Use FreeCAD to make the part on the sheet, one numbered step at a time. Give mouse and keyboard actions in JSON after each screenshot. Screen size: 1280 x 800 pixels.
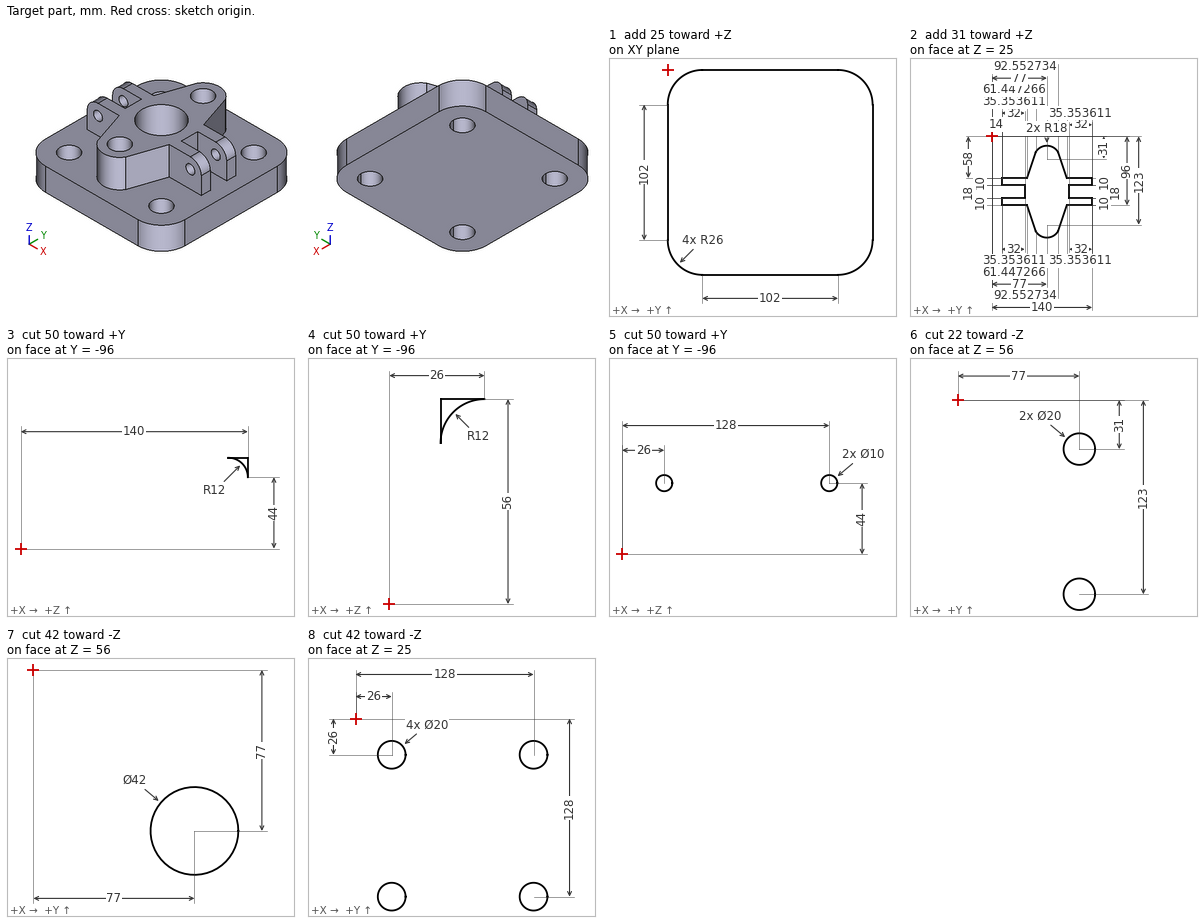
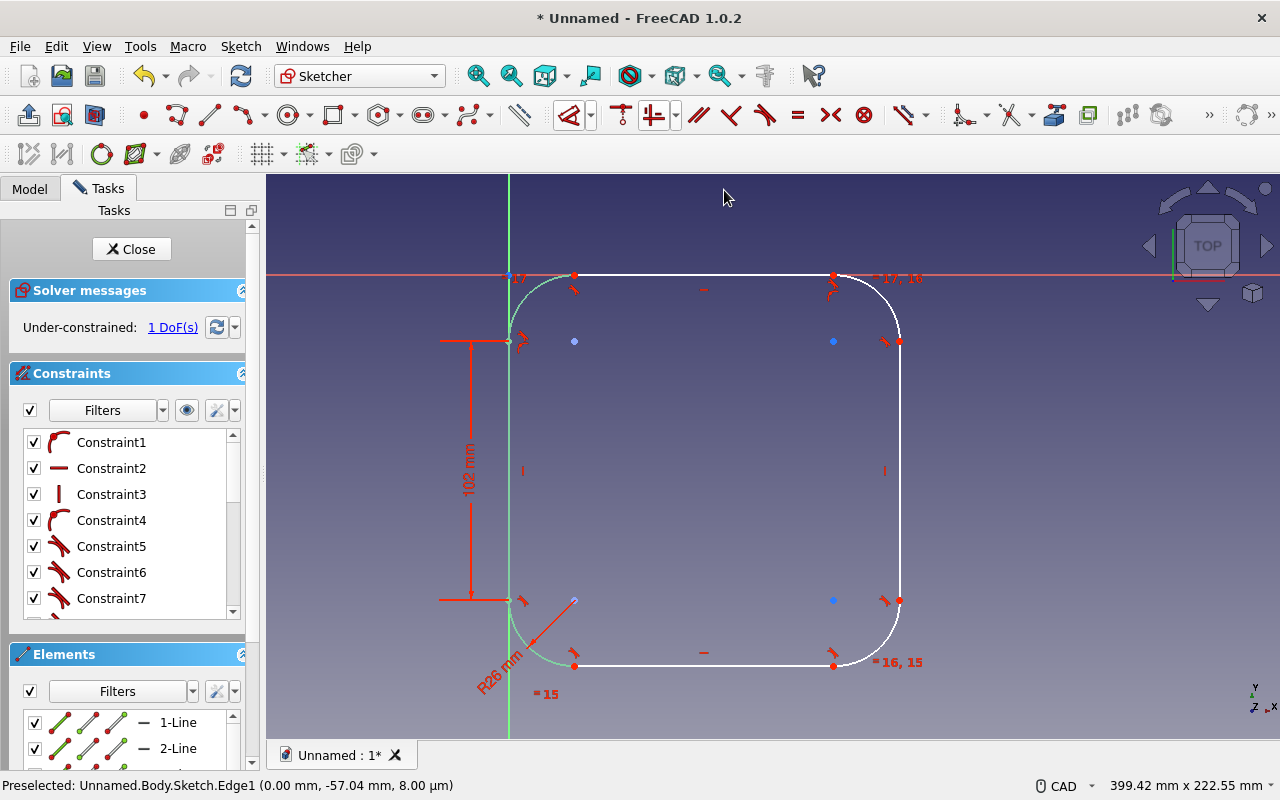
{"action": "left_click", "coordinate": [653, 666]}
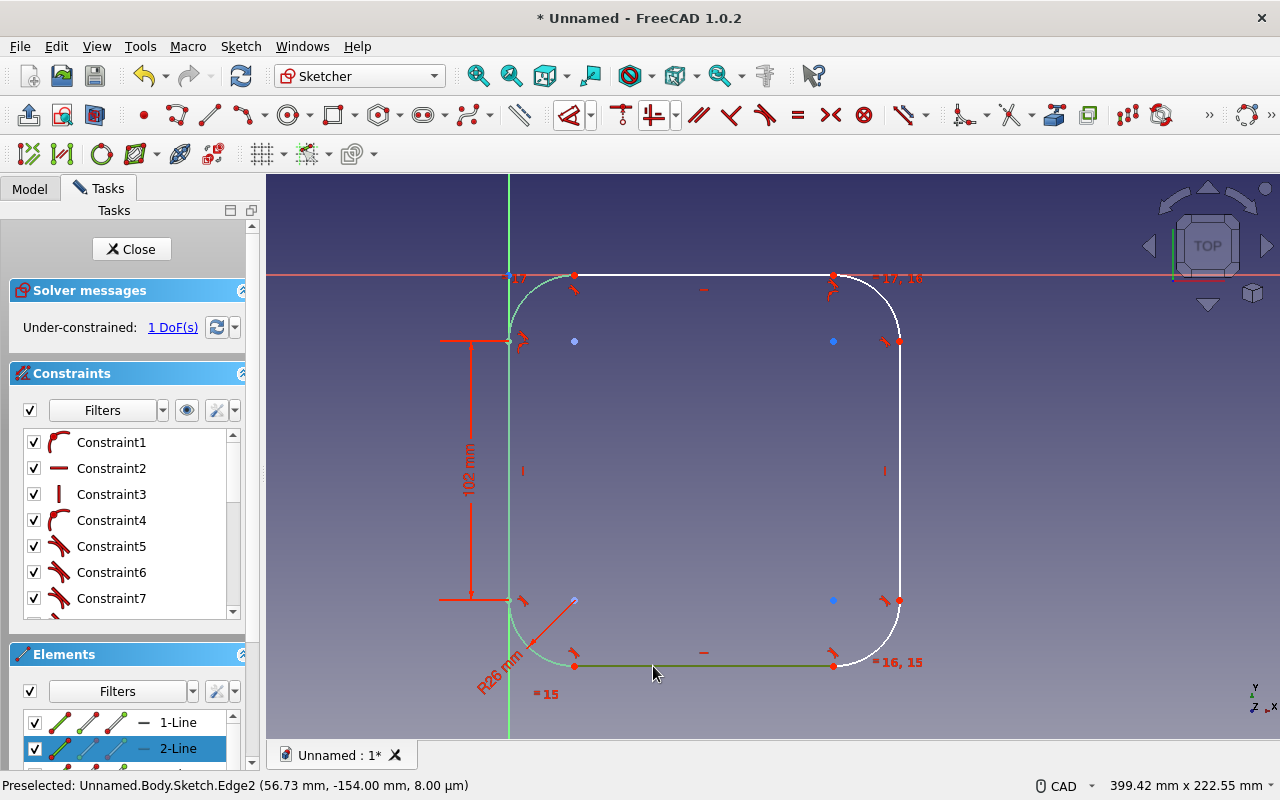
{"action": "key", "text": "l"}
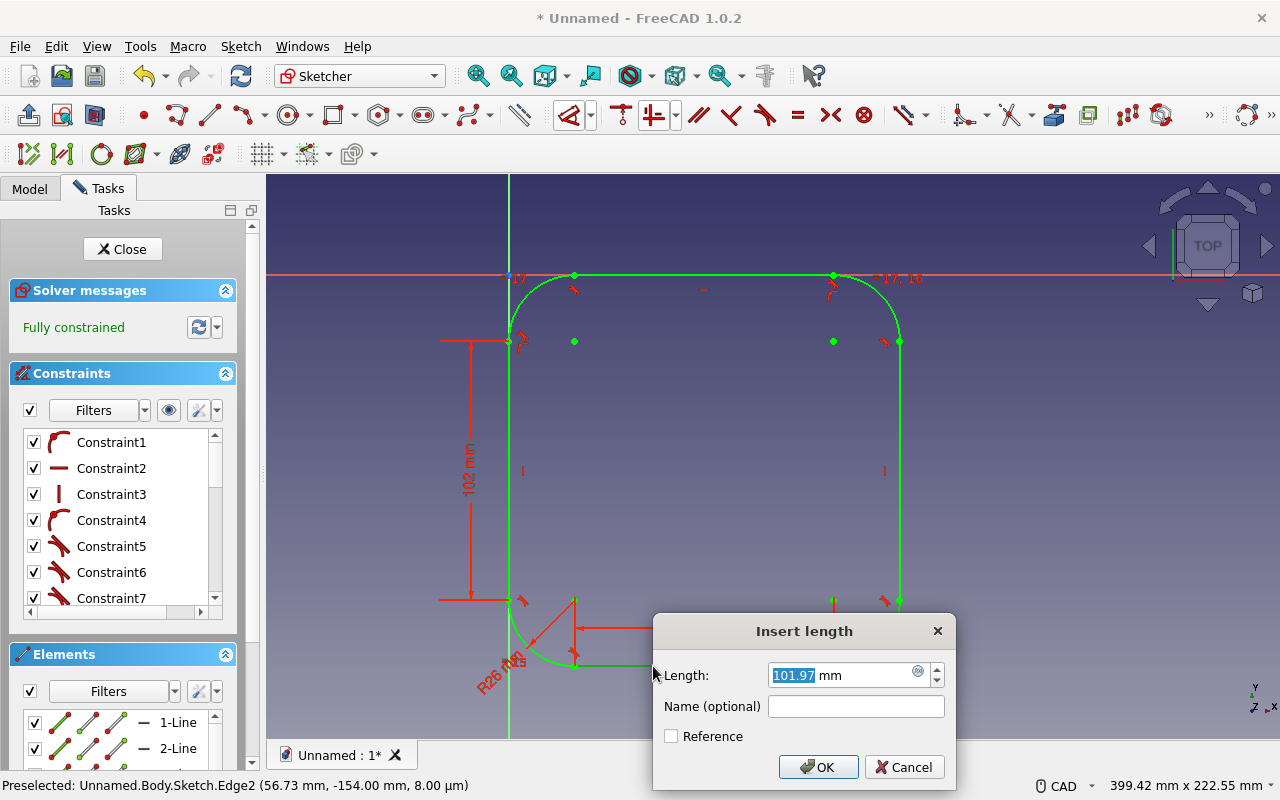
{"action": "type", "text": "102"}
{"action": "key", "text": "Return"}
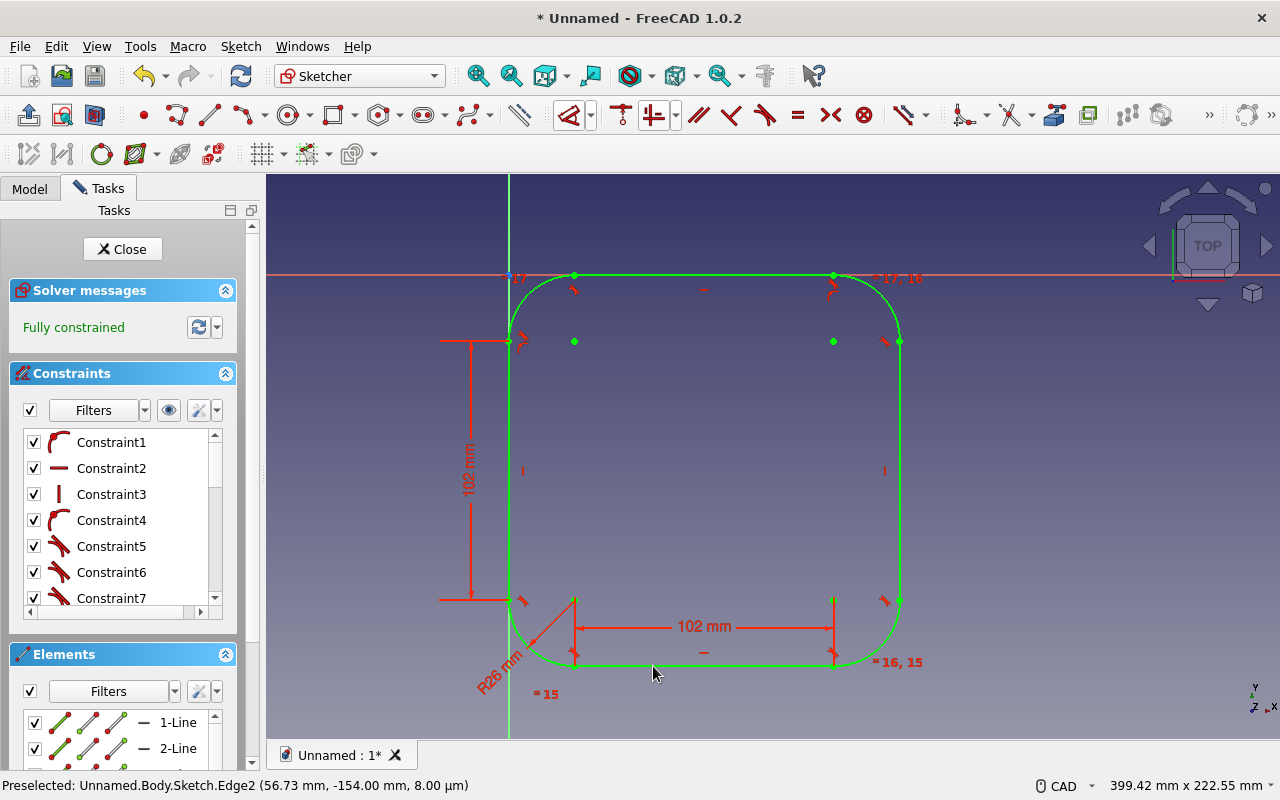
{"action": "left_click", "coordinate": [123, 249]}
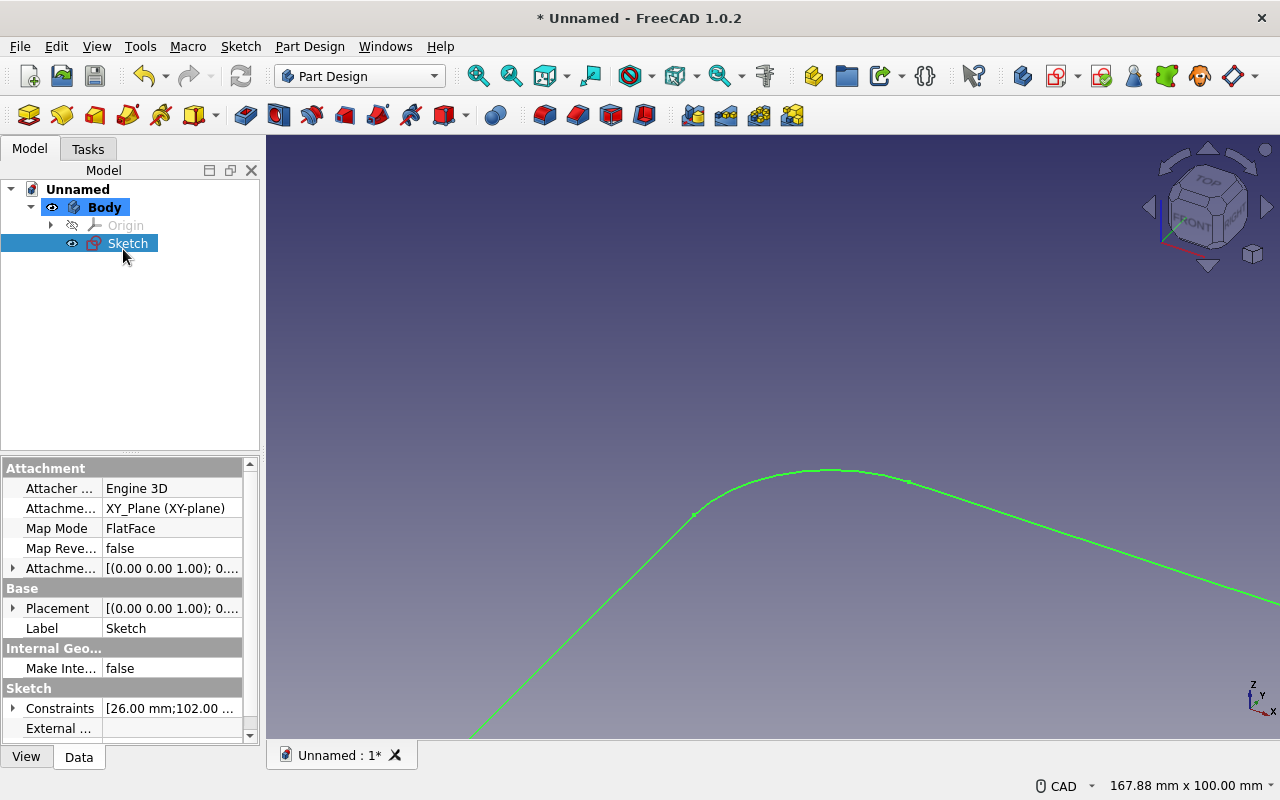
{"action": "left_click", "coordinate": [29, 116]}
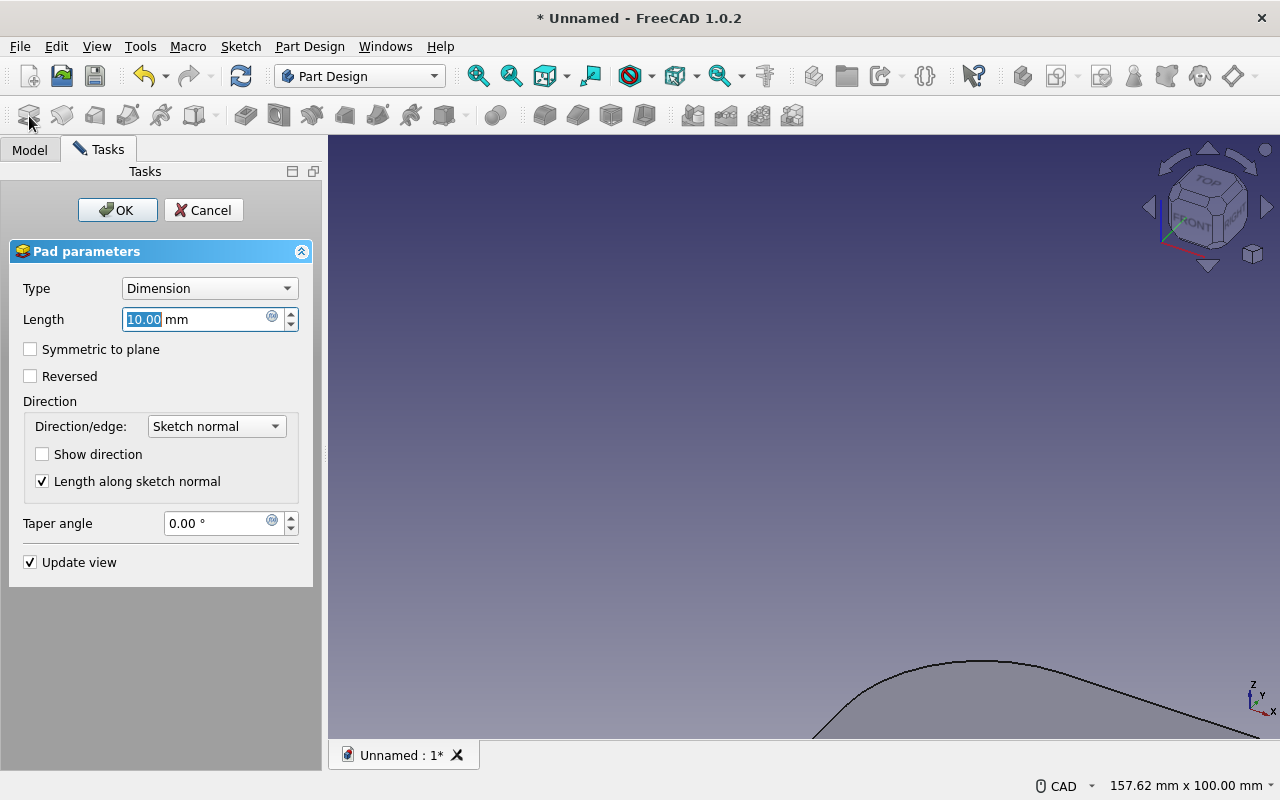
{"action": "type", "text": "25"}
{"action": "key", "text": "Tab"}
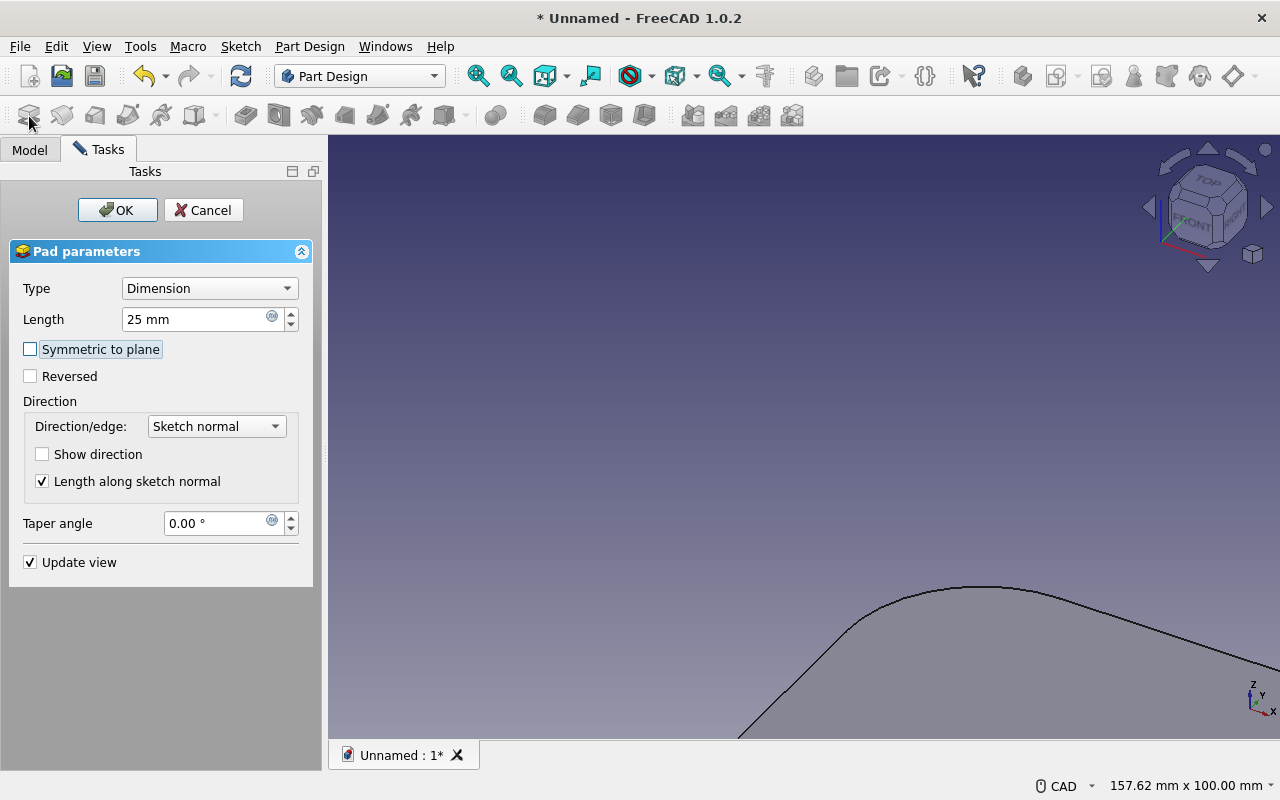
{"action": "left_click", "coordinate": [118, 210]}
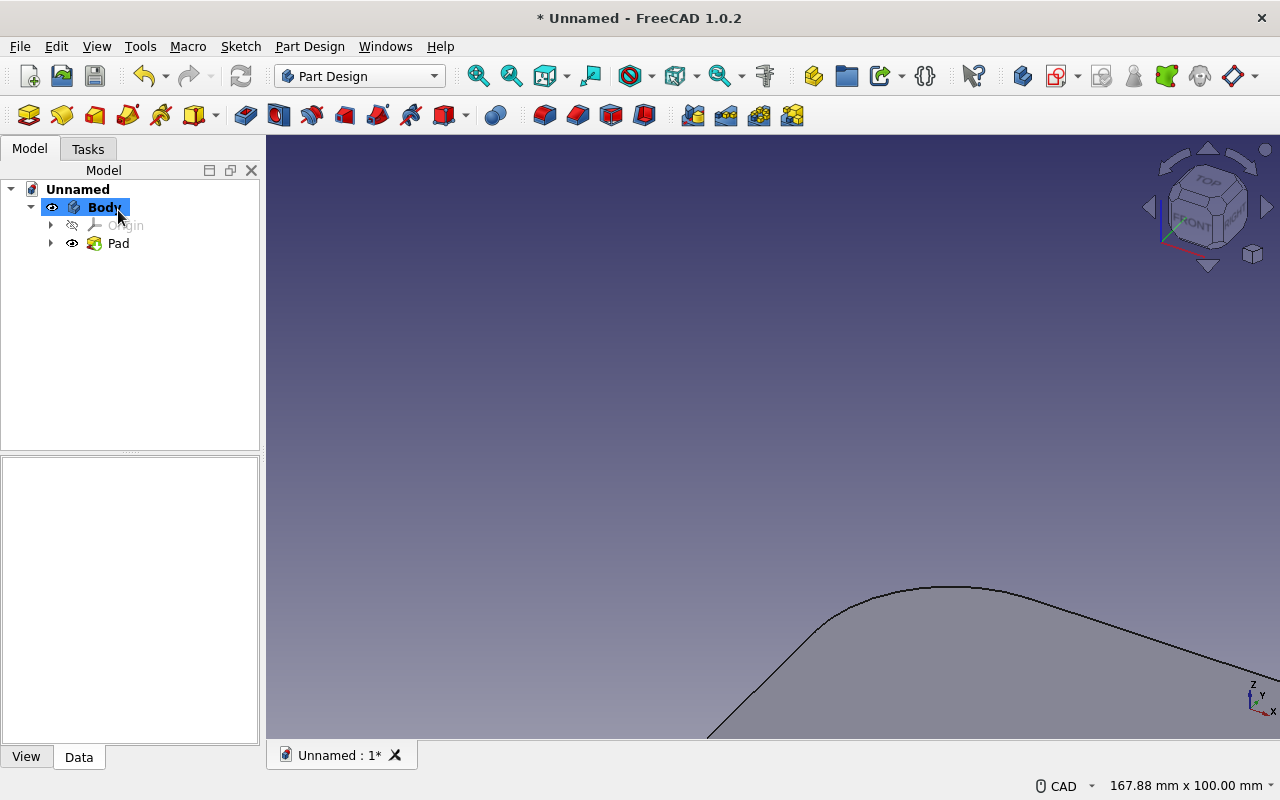
{"action": "left_click", "coordinate": [479, 76]}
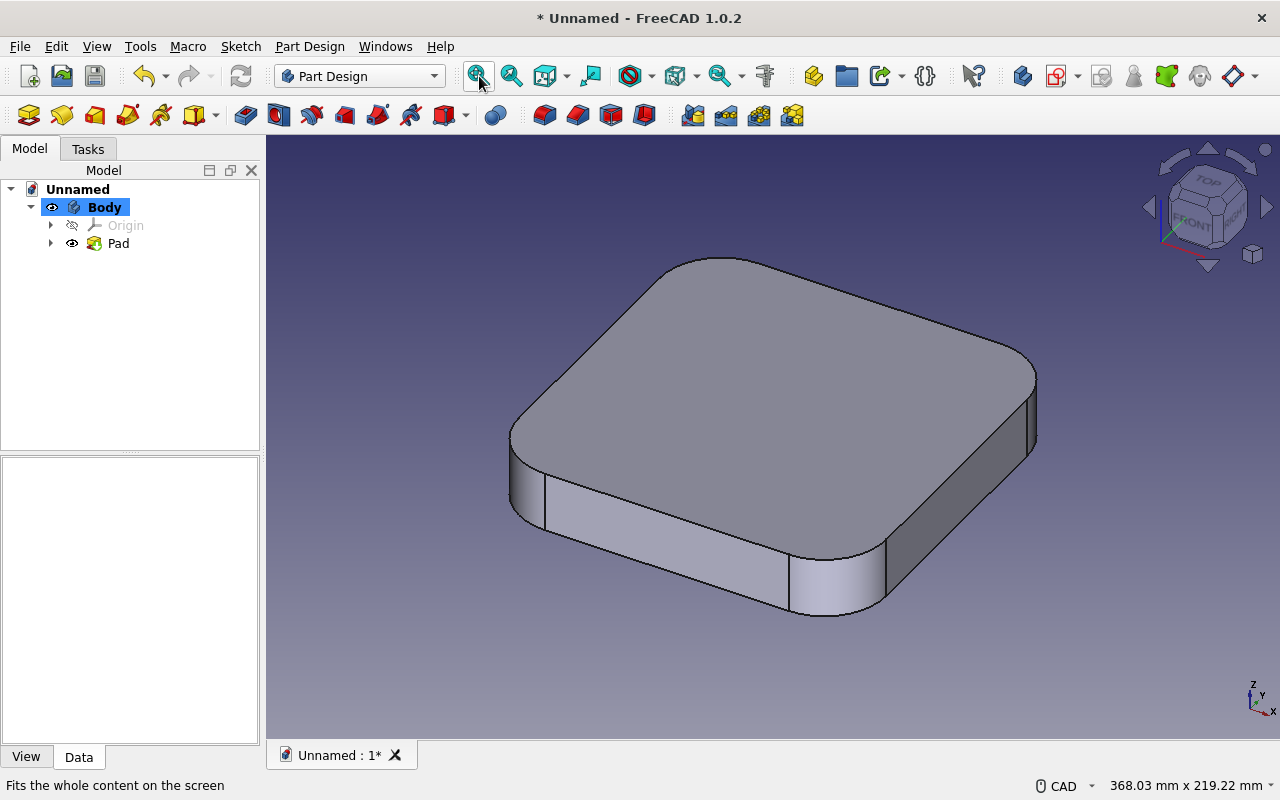
{"action": "left_click", "coordinate": [773, 408]}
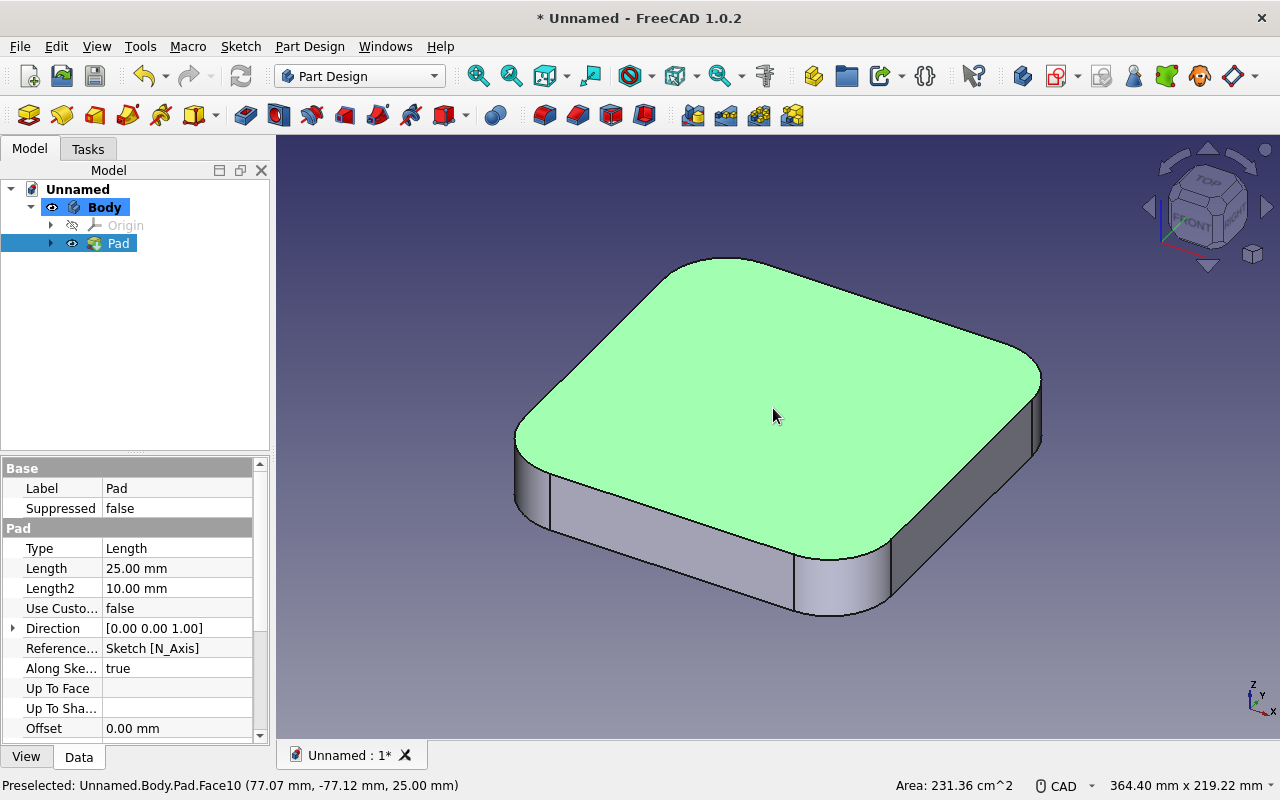
{"action": "left_click", "coordinate": [1056, 76]}